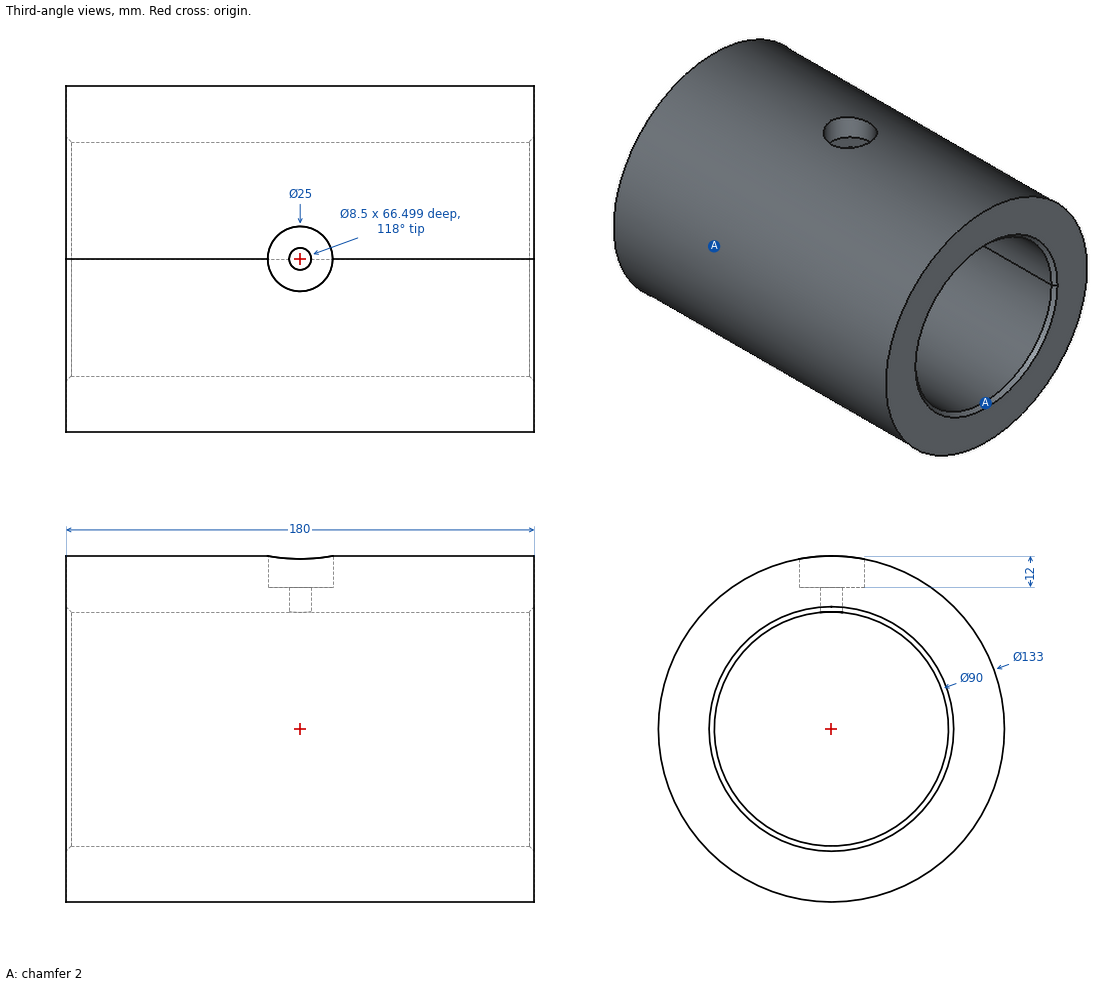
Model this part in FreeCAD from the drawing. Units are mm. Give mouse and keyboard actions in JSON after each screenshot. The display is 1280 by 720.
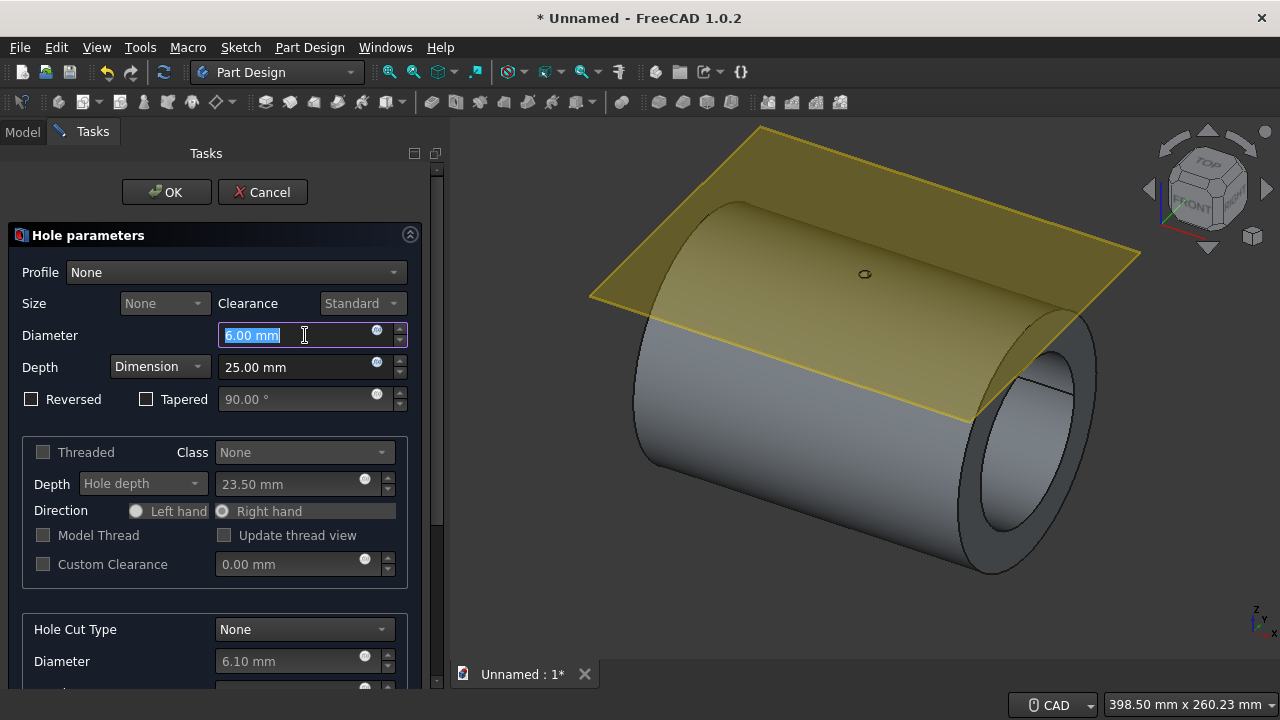
{"action": "type", "text": "8.5"}
{"action": "key", "text": "Tab"}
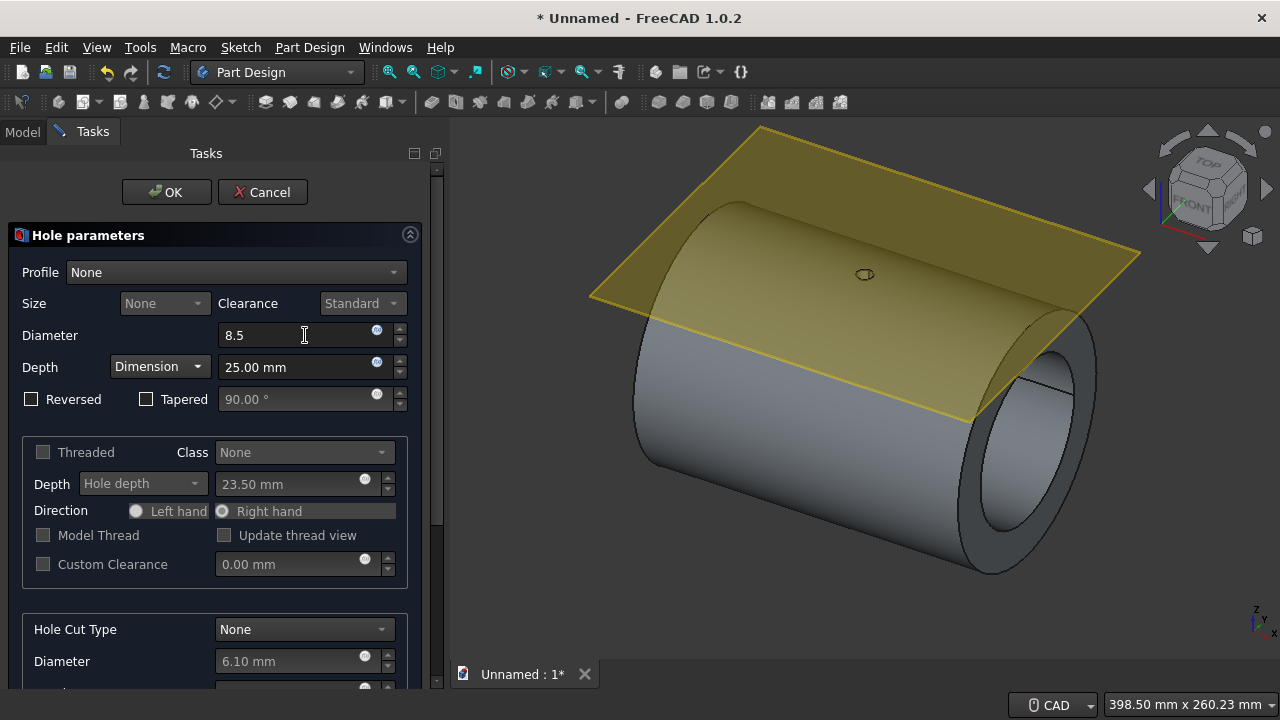
{"action": "triple_click", "coordinate": [305, 367]}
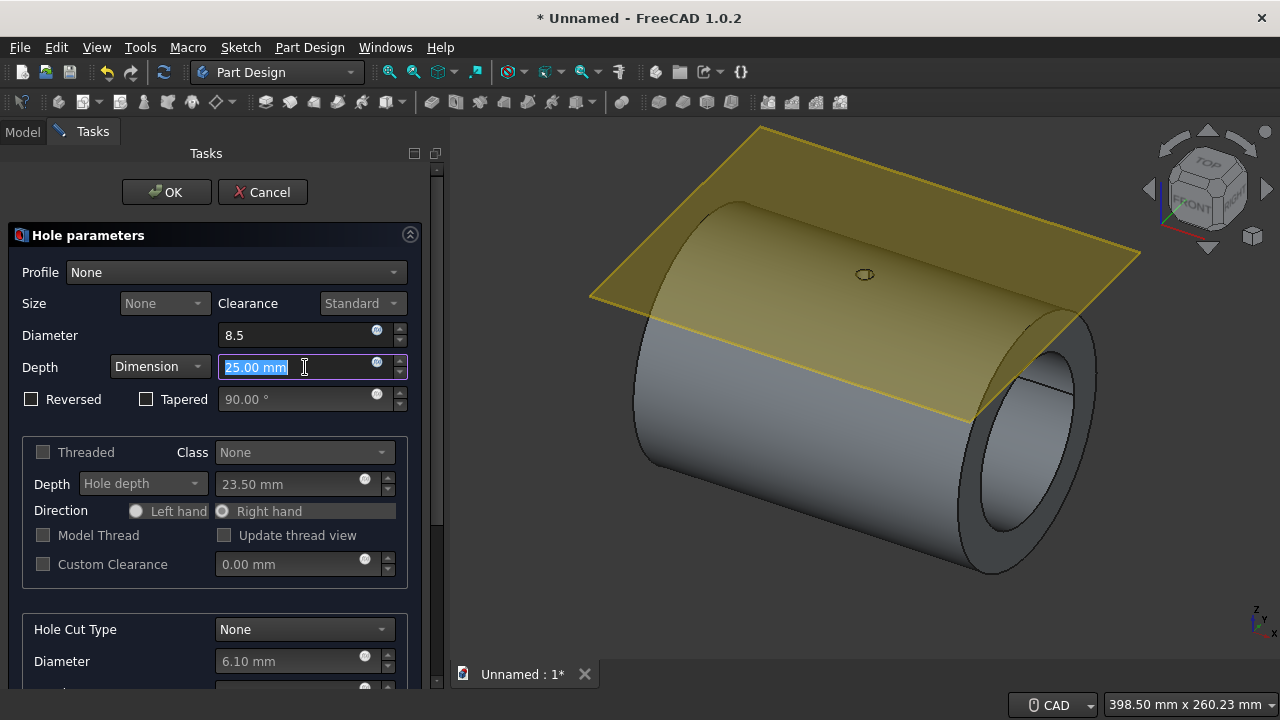
{"action": "type", "text": "66.499"}
{"action": "key", "text": "Tab"}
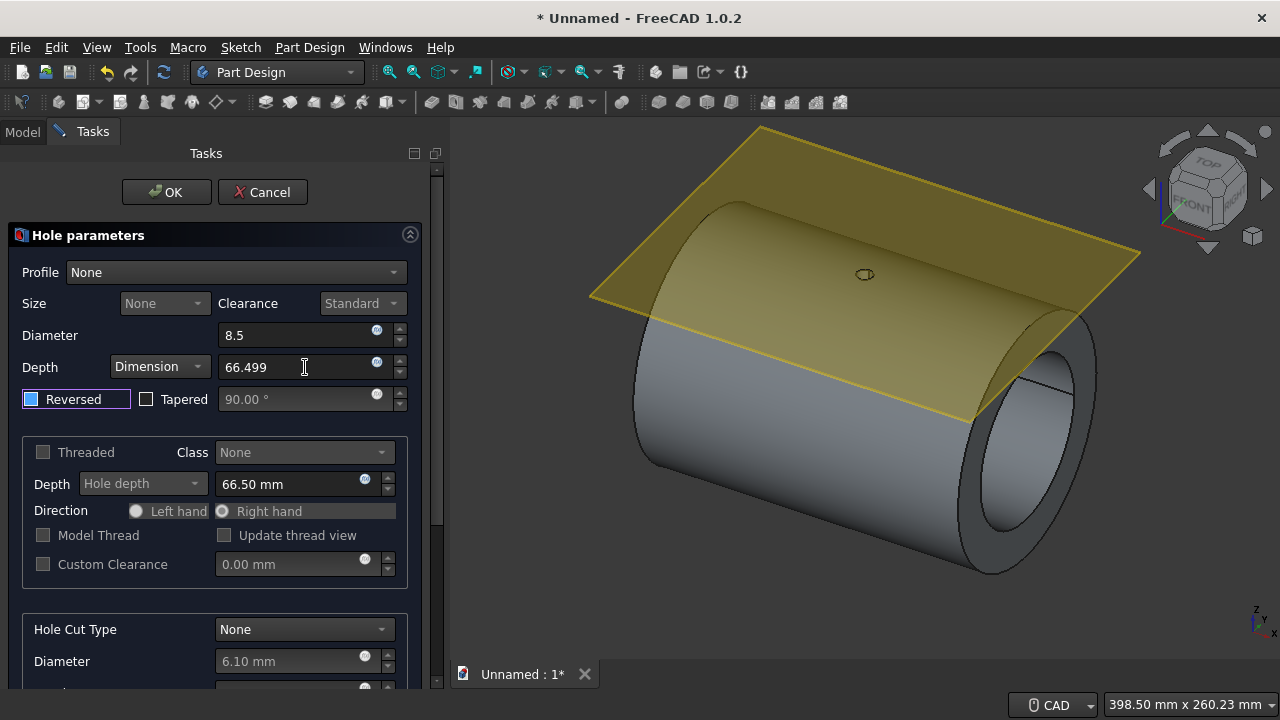
{"action": "left_click", "coordinate": [167, 192]}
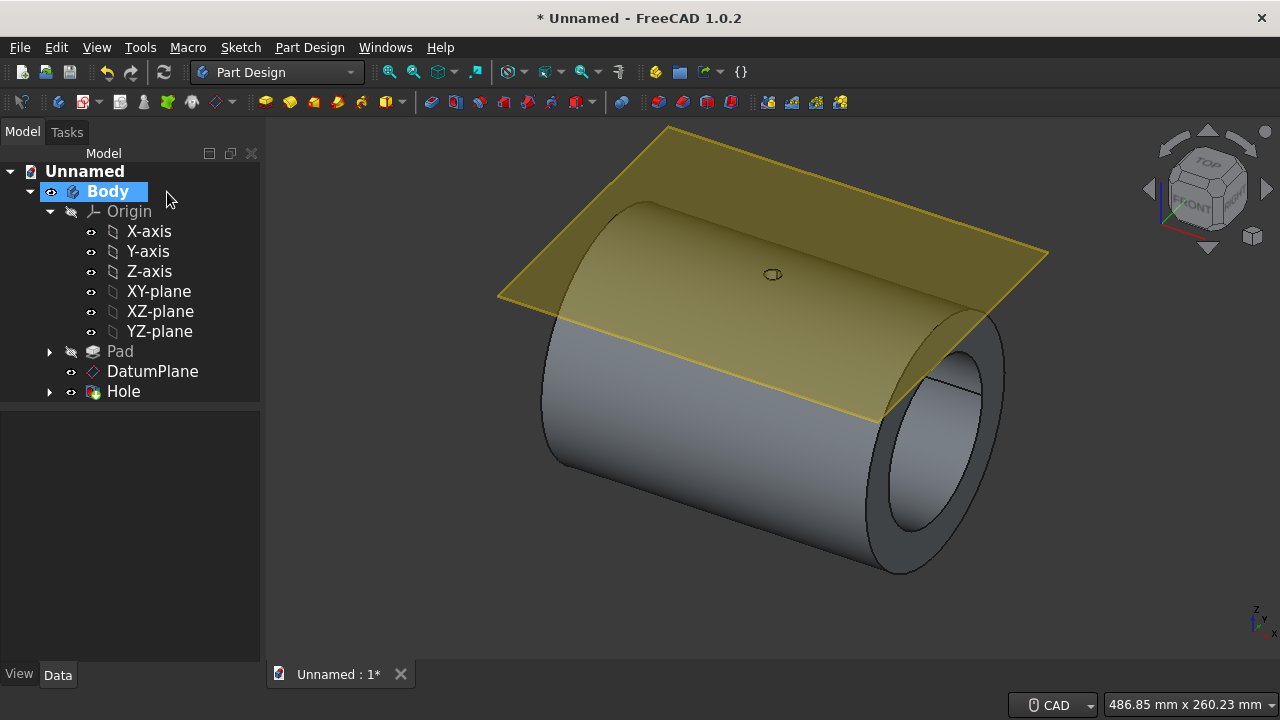
{"action": "left_click", "coordinate": [116, 372]}
{"action": "key", "text": "space"}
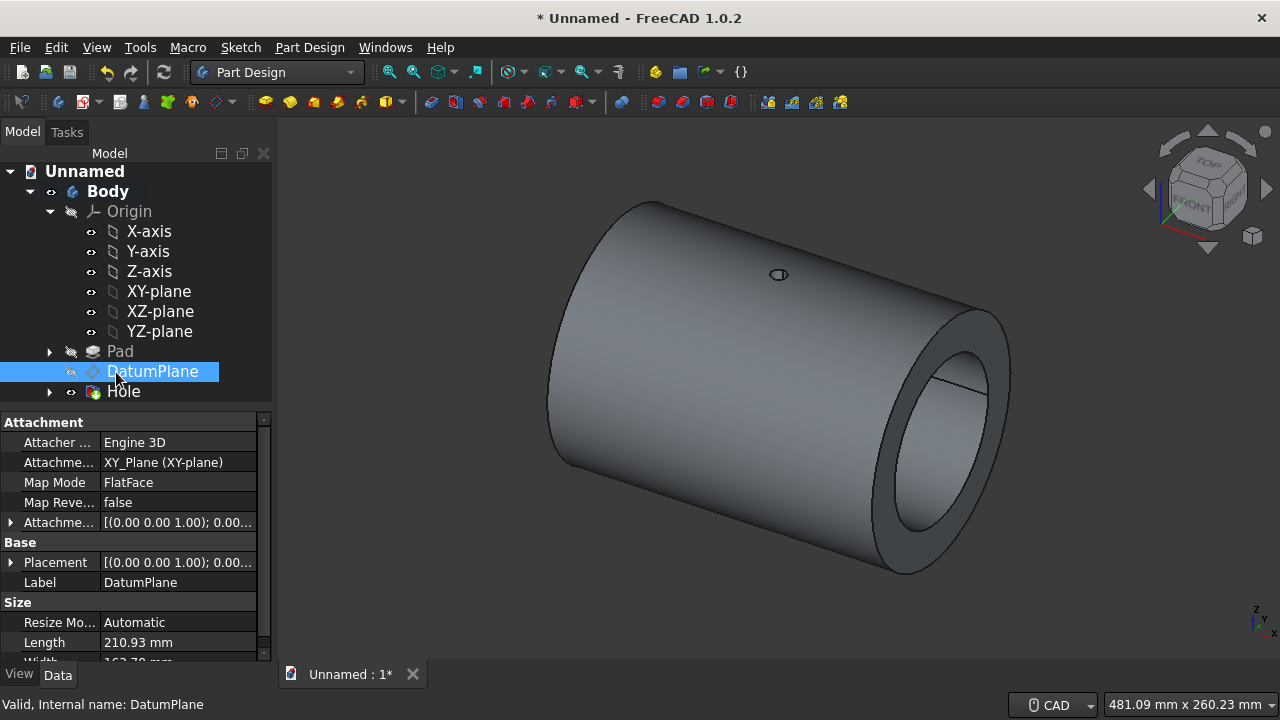
{"action": "left_click", "coordinate": [136, 292]}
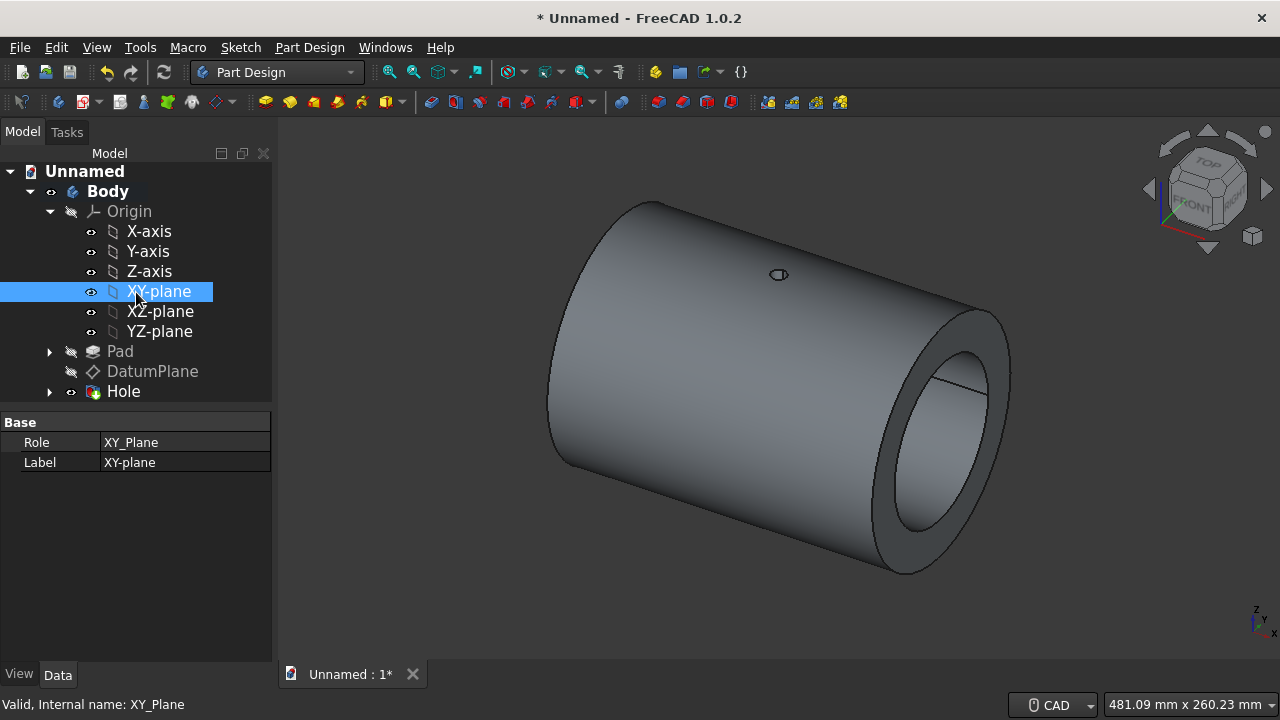
{"action": "left_click", "coordinate": [216, 102]}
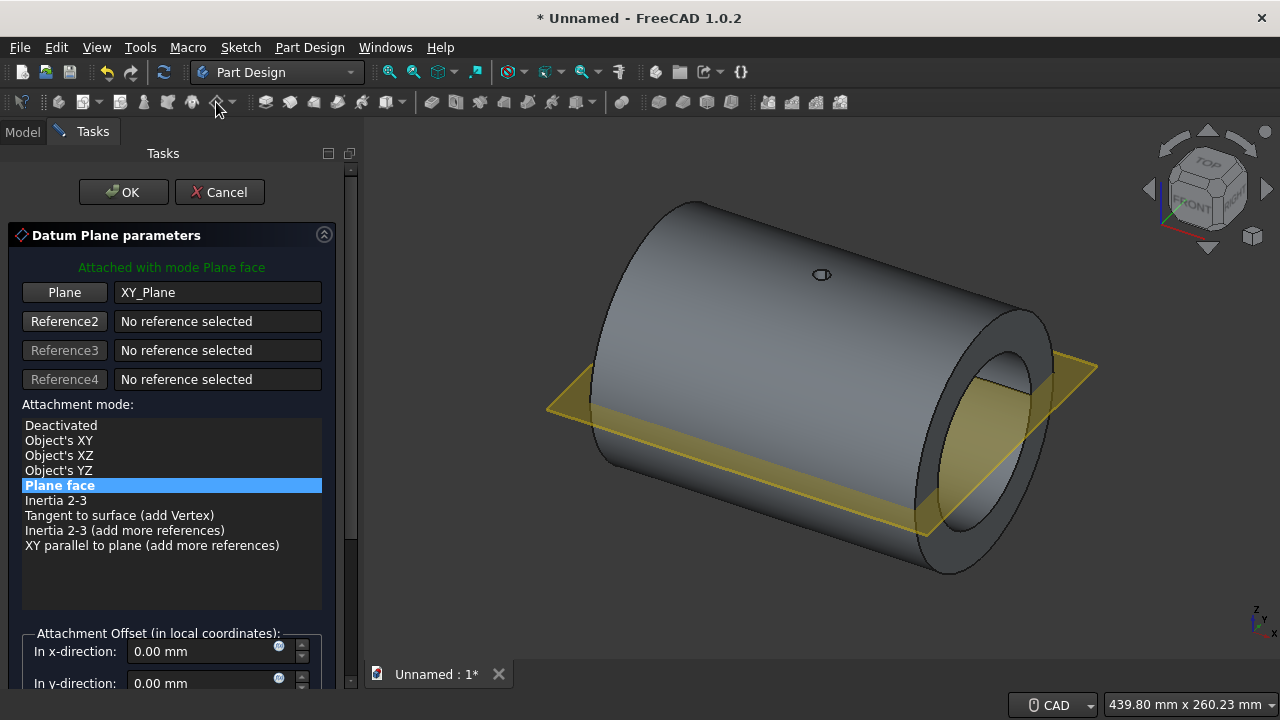
{"action": "scroll", "coordinate": [351, 426], "scroll_direction": "down", "scroll_amount": 2}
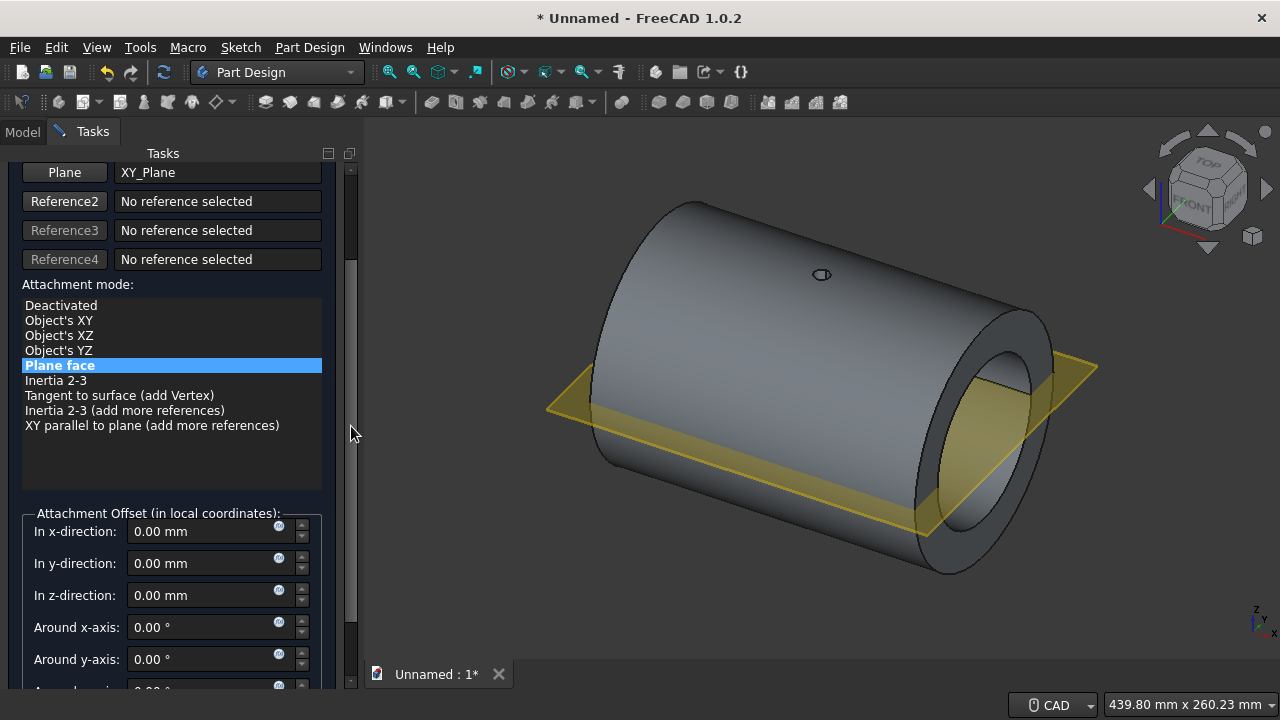
{"action": "triple_click", "coordinate": [210, 595]}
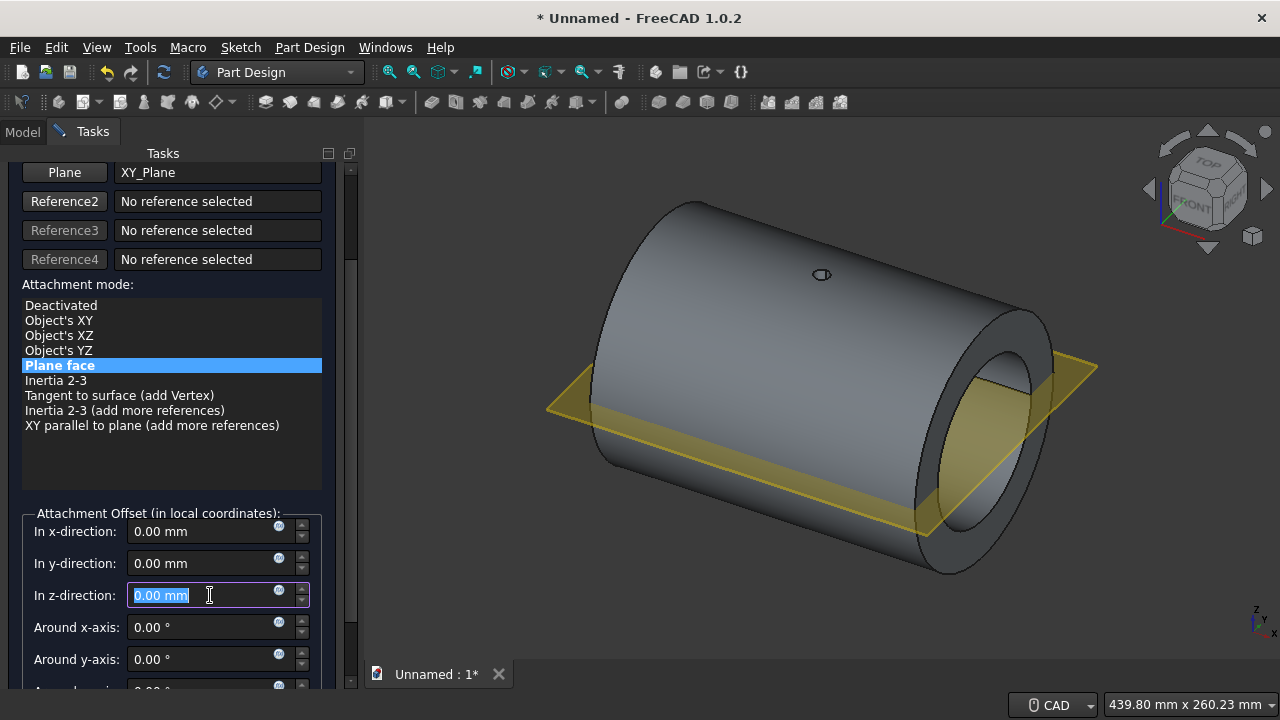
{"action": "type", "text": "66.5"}
{"action": "key", "text": "Tab"}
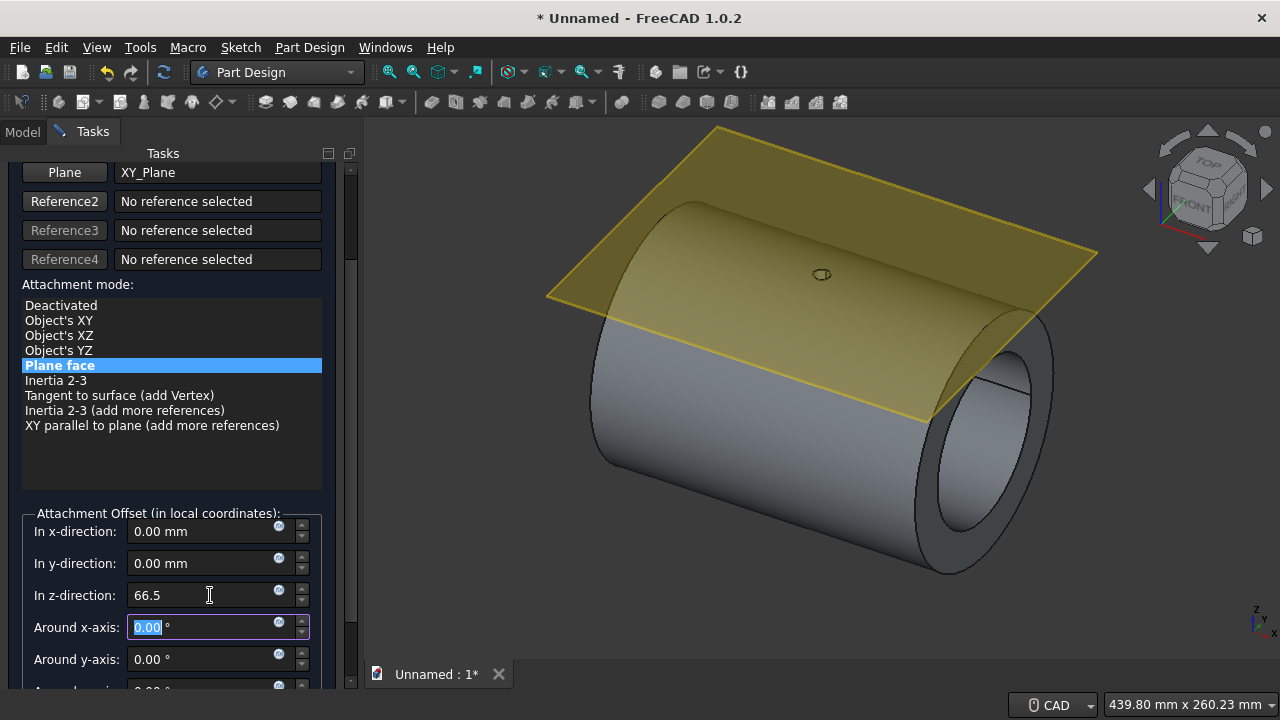
{"action": "scroll", "coordinate": [351, 426], "scroll_direction": "up", "scroll_amount": 3}